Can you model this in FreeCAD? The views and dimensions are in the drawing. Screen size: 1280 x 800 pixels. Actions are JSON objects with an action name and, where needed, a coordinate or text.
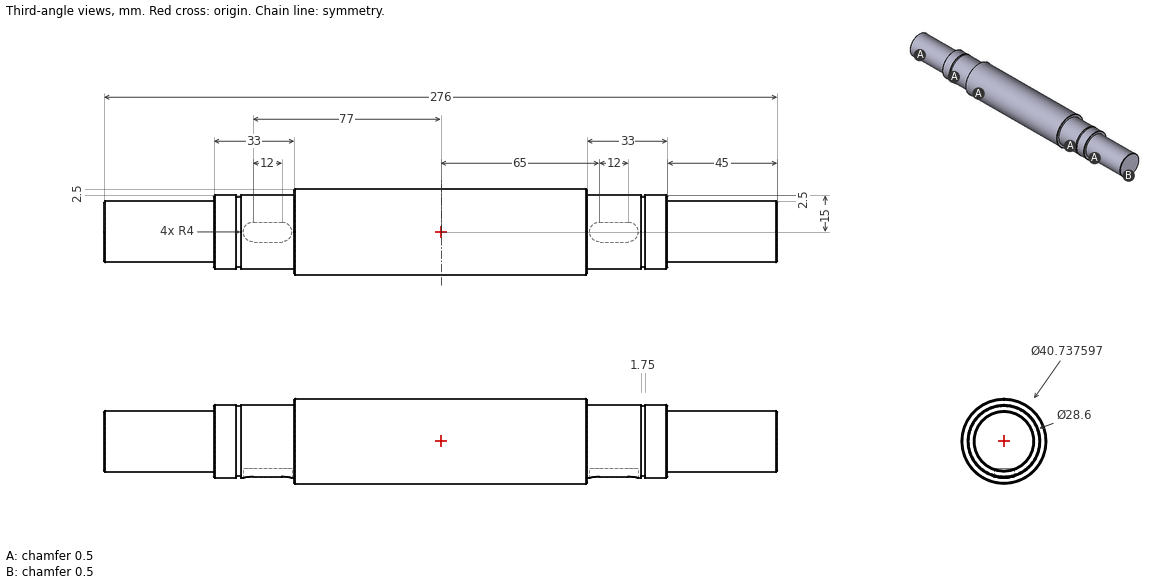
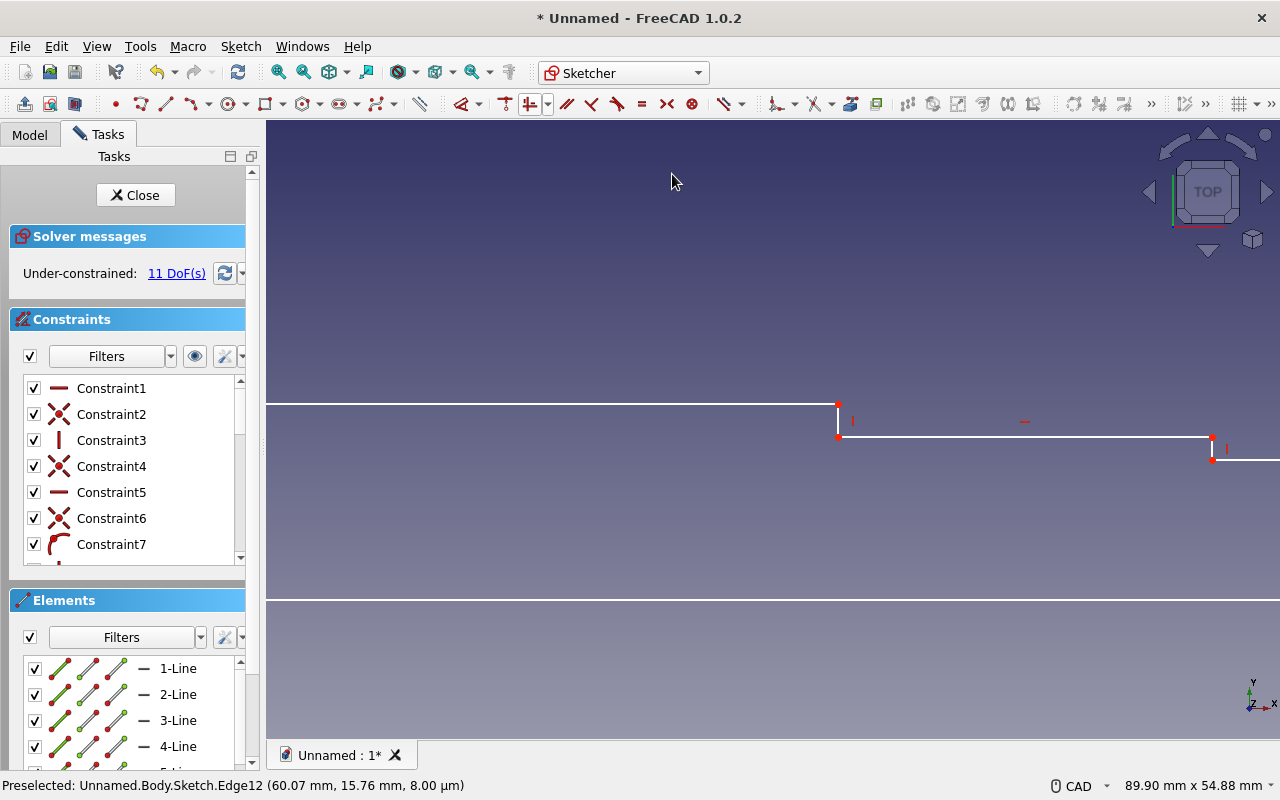
{"action": "scroll", "coordinate": [842, 411], "scroll_direction": "down", "scroll_amount": 8}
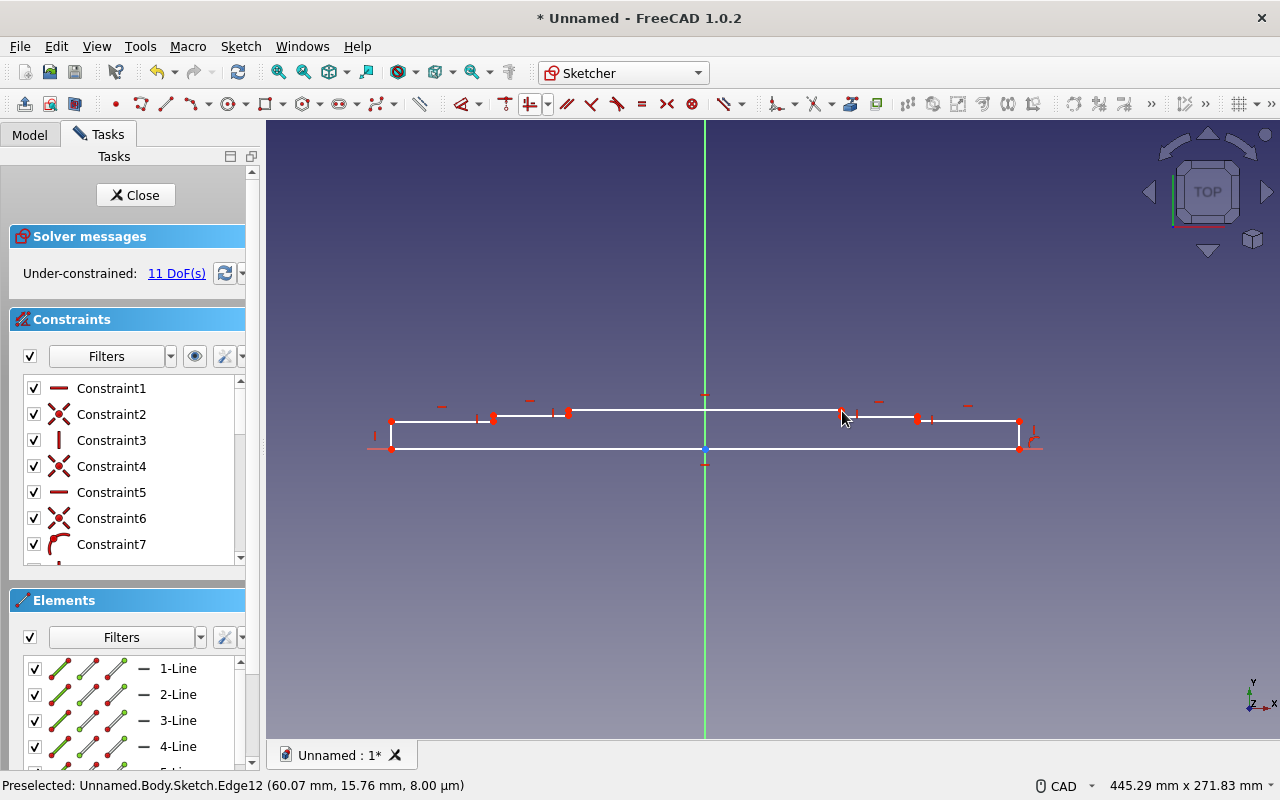
{"action": "left_click", "coordinate": [1019, 421]}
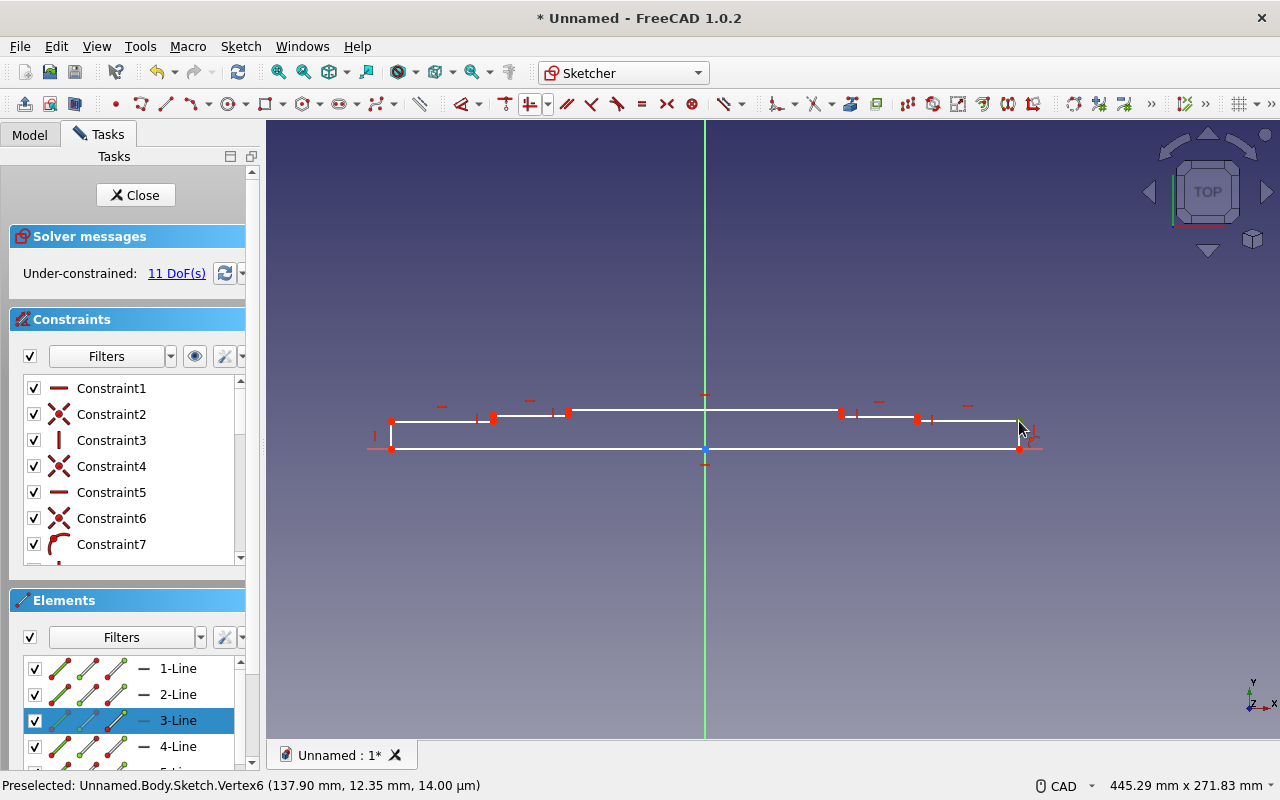
{"action": "left_click", "coordinate": [391, 422]}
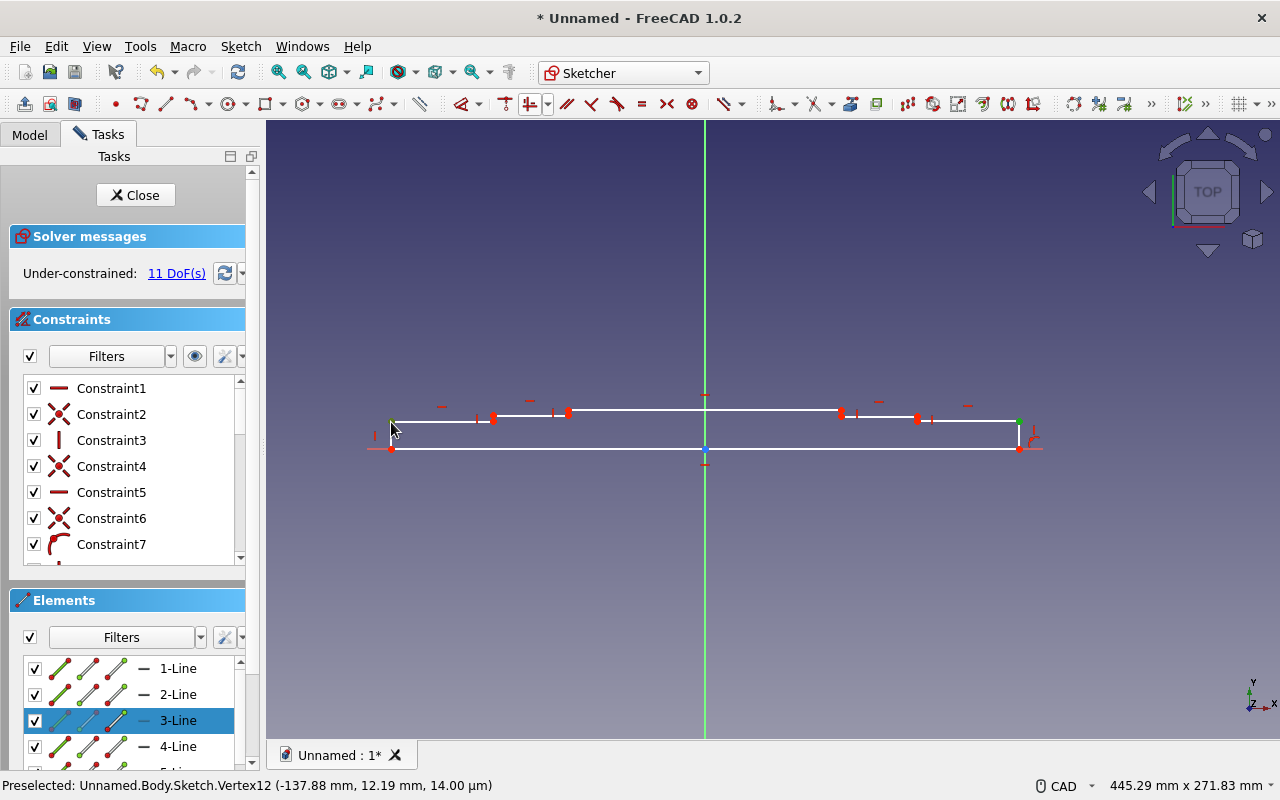
{"action": "left_click", "coordinate": [705, 671]}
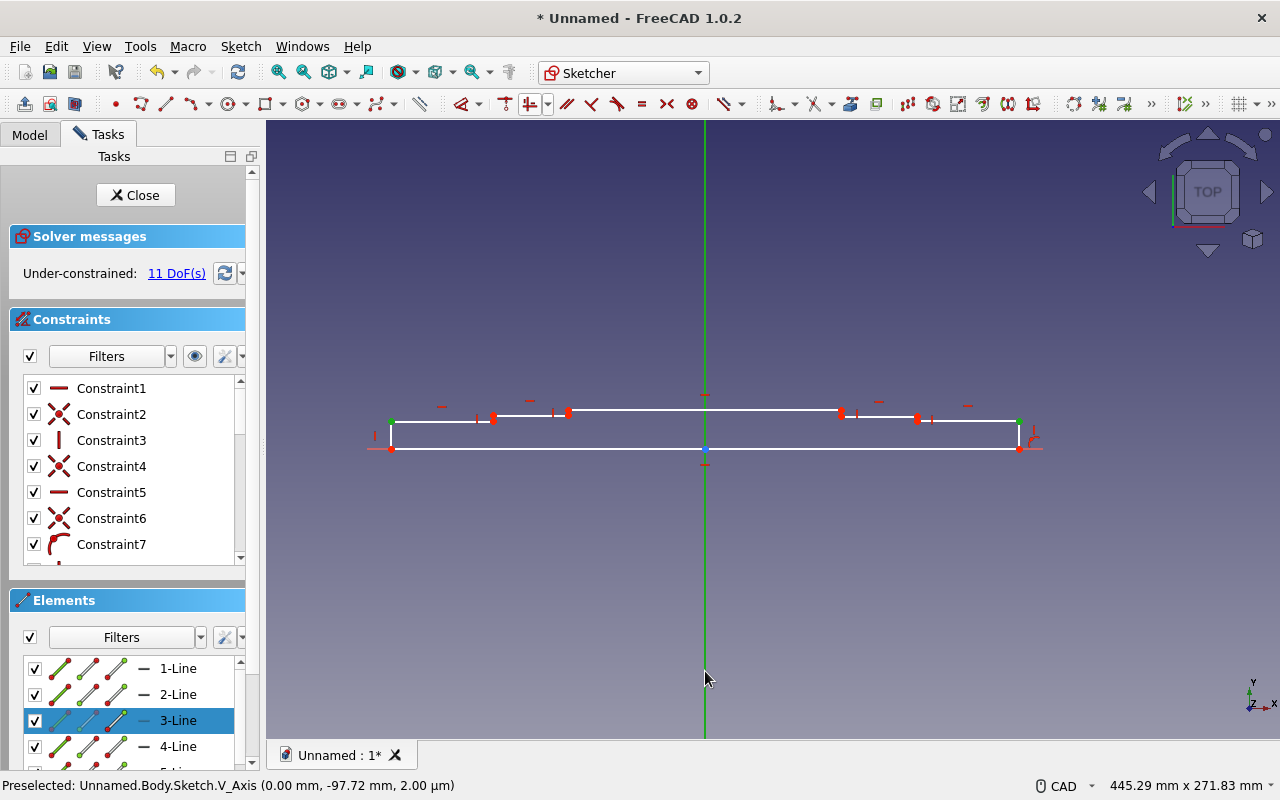
{"action": "left_click", "coordinate": [667, 104]}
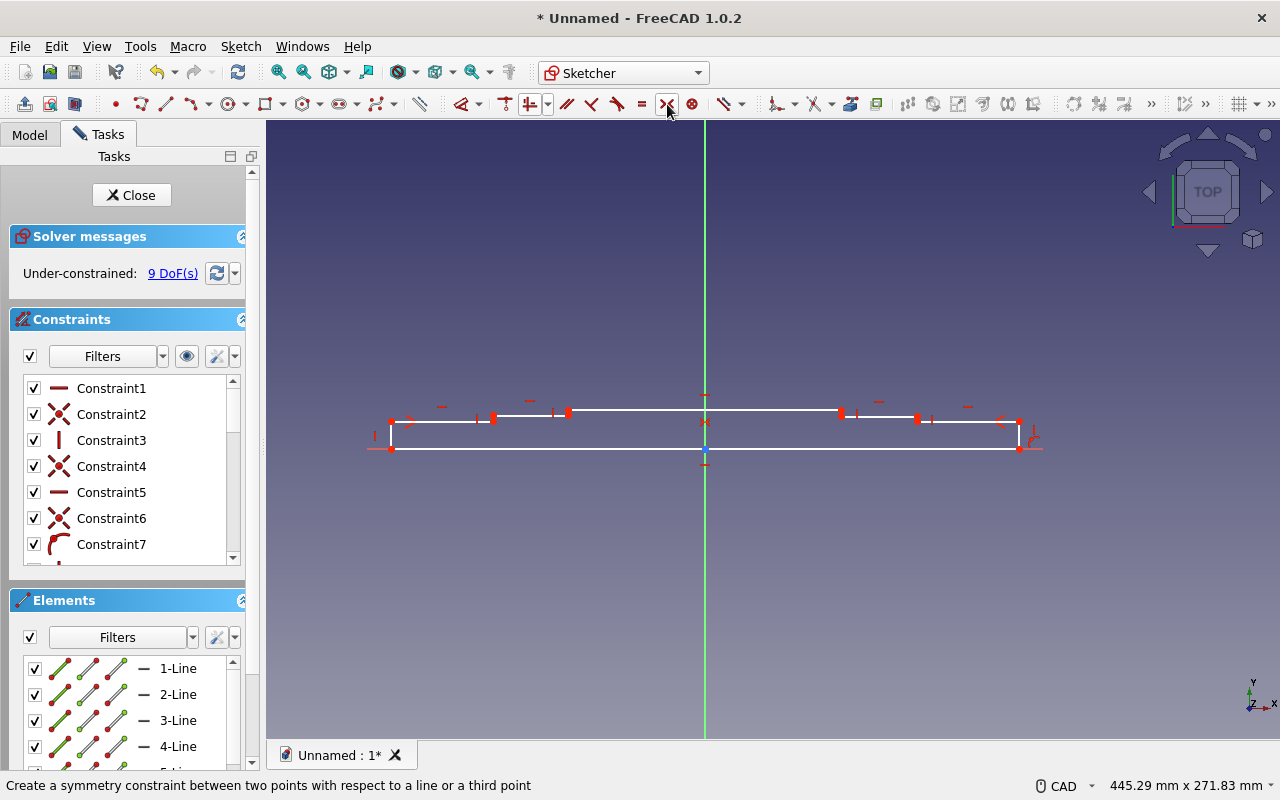
{"action": "scroll", "coordinate": [917, 417], "scroll_direction": "up", "scroll_amount": 5}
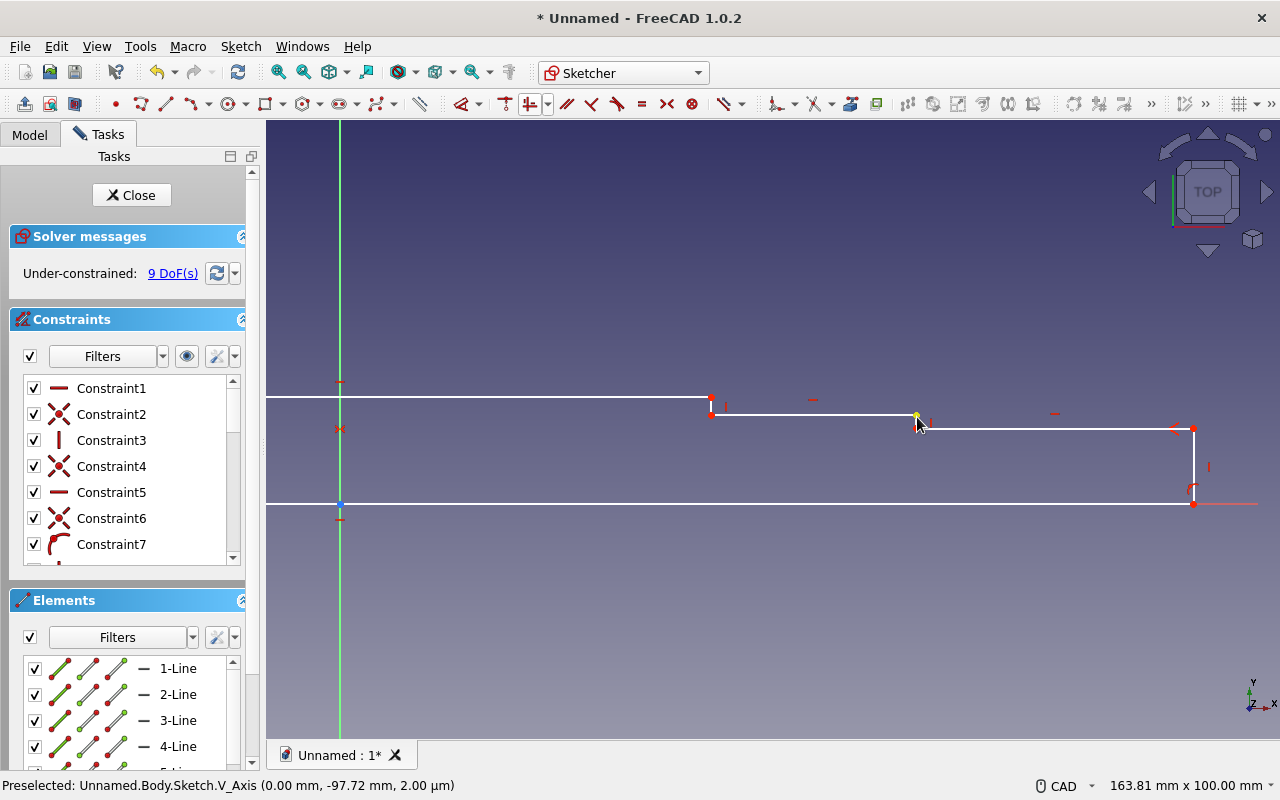
{"action": "left_click", "coordinate": [916, 415]}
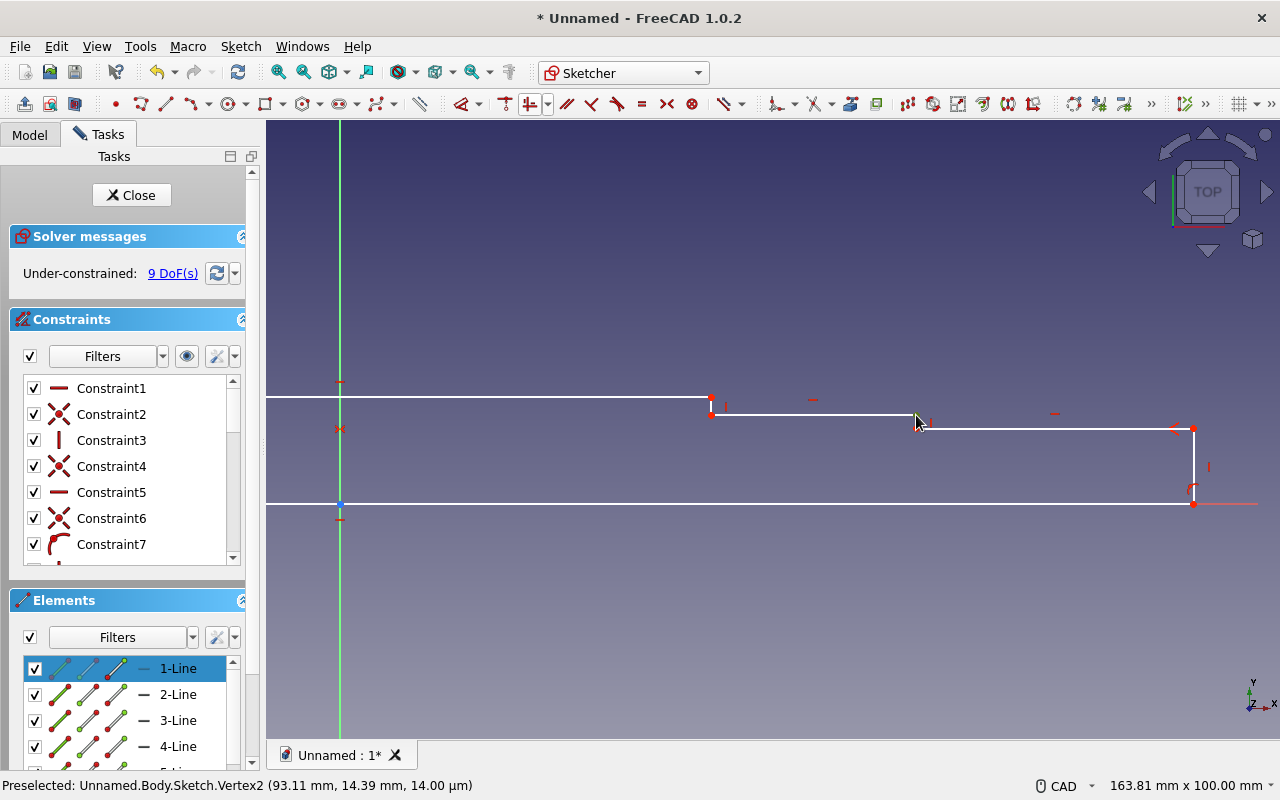
{"action": "scroll", "coordinate": [917, 417], "scroll_direction": "down", "scroll_amount": 5}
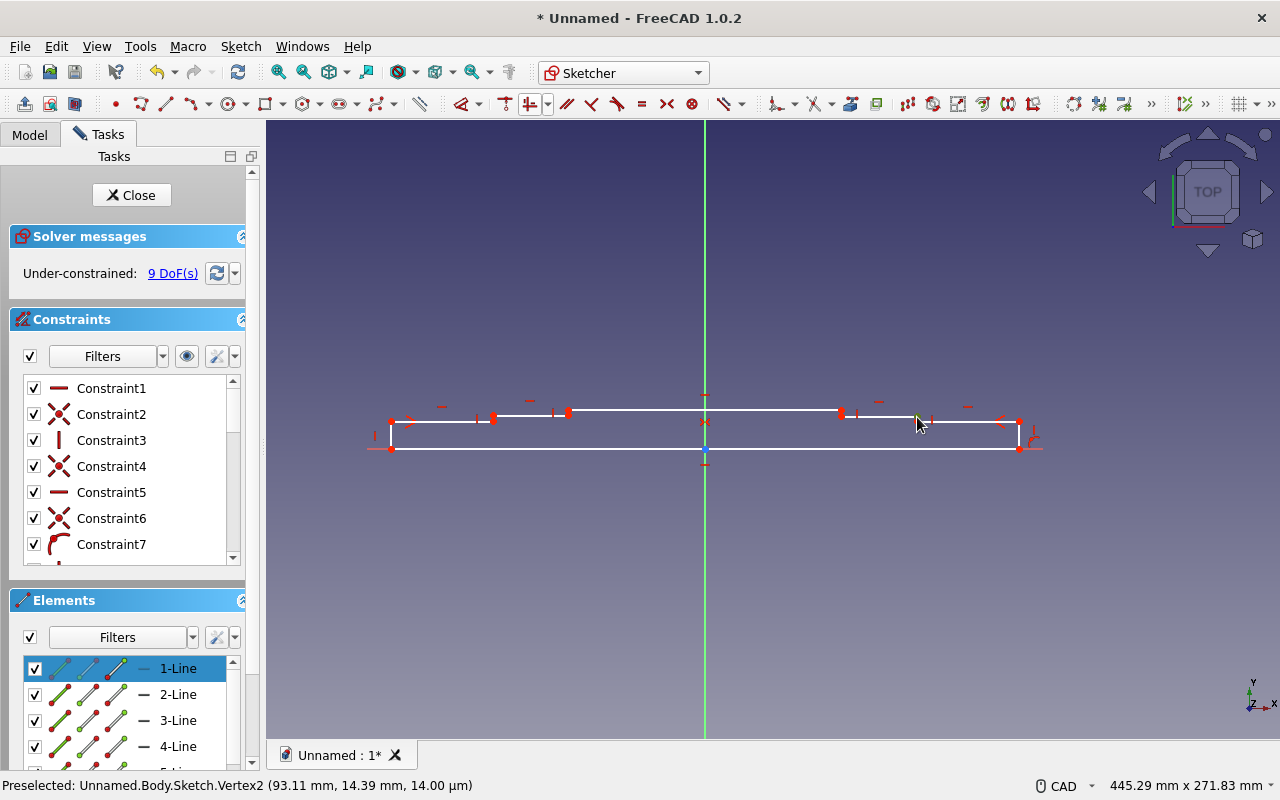
{"action": "scroll", "coordinate": [493, 416], "scroll_direction": "up", "scroll_amount": 4}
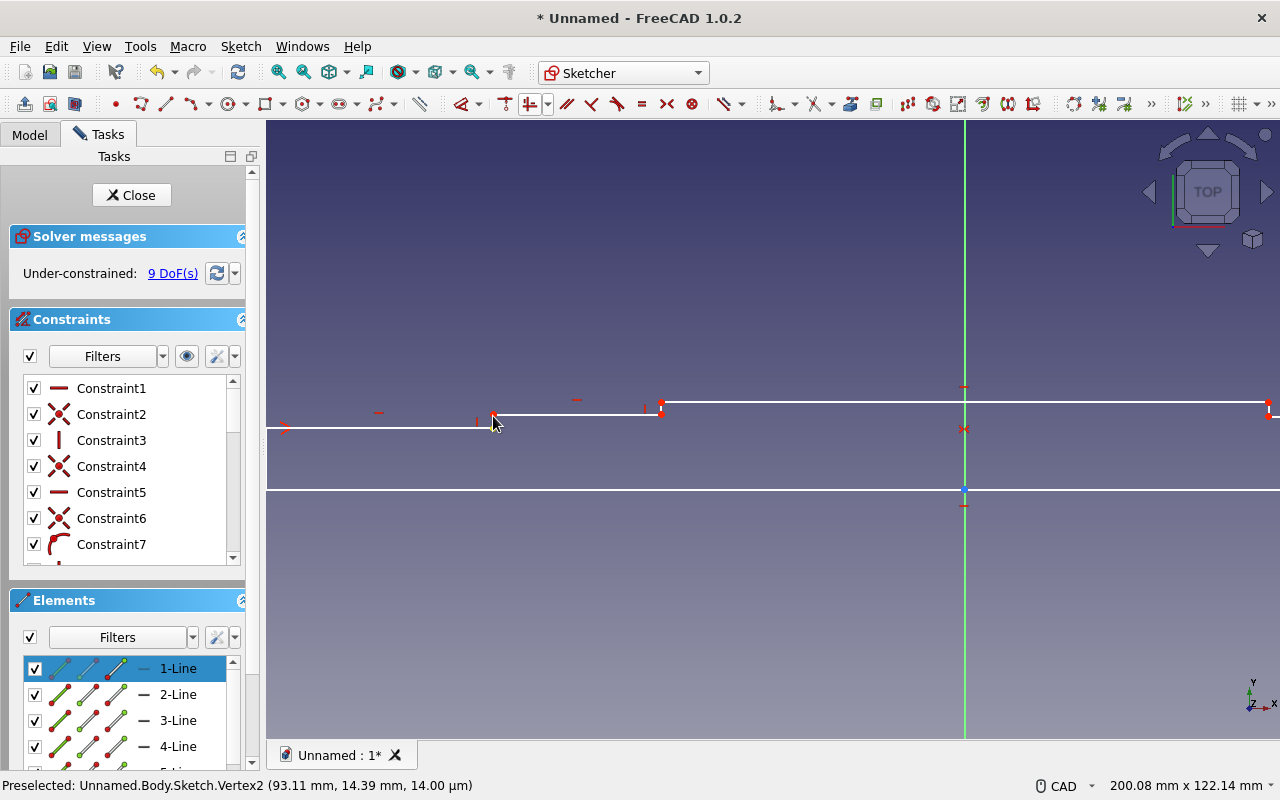
{"action": "left_click", "coordinate": [493, 415]}